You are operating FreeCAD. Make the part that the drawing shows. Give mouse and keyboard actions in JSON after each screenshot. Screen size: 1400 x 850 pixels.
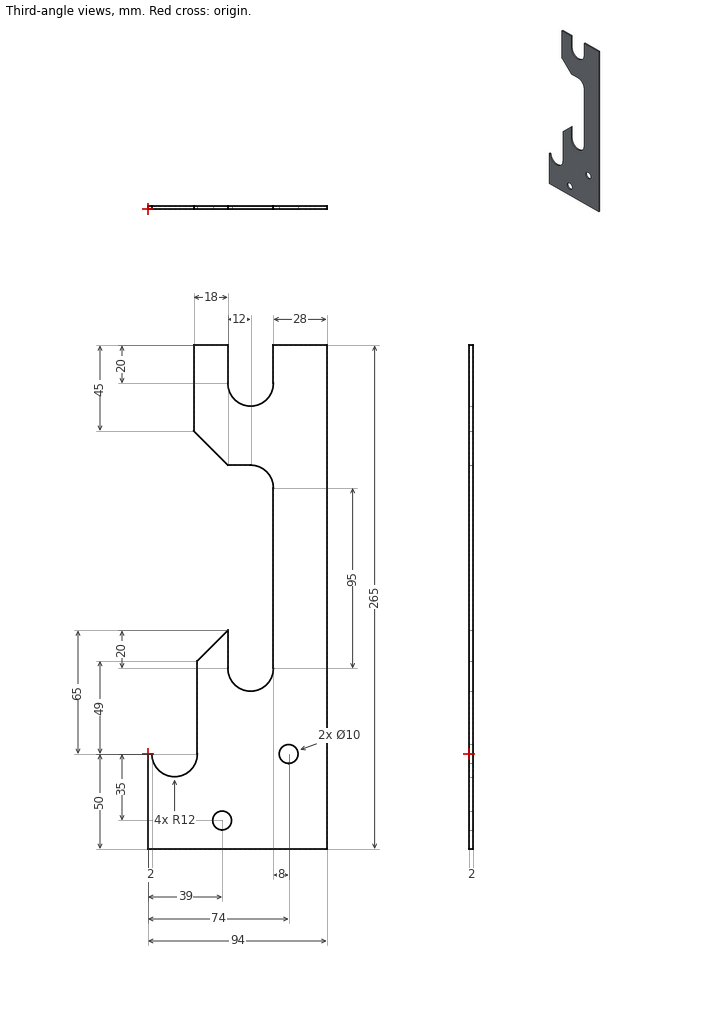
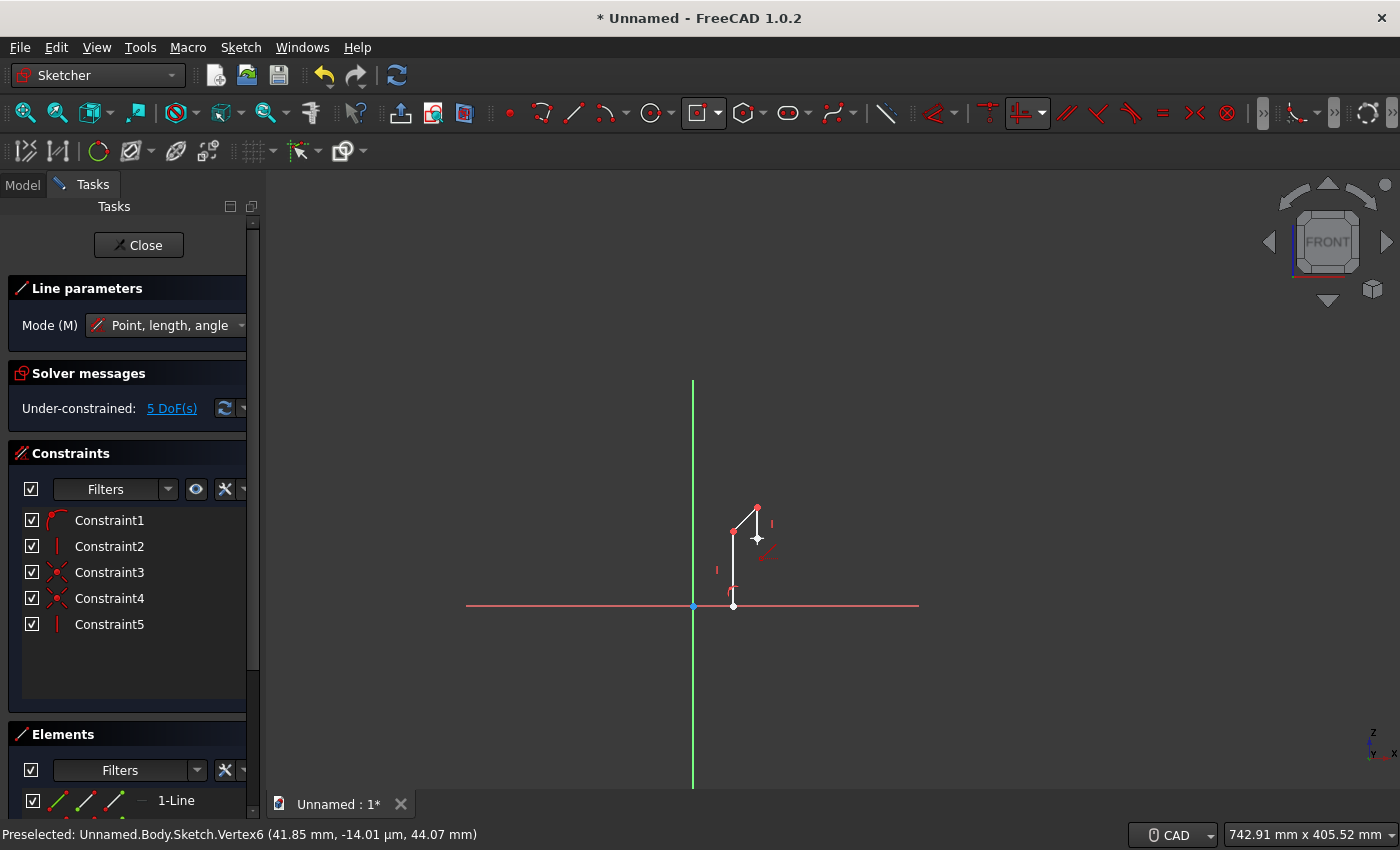
{"action": "left_click", "coordinate": [794, 538]}
{"action": "left_click", "coordinate": [794, 393]}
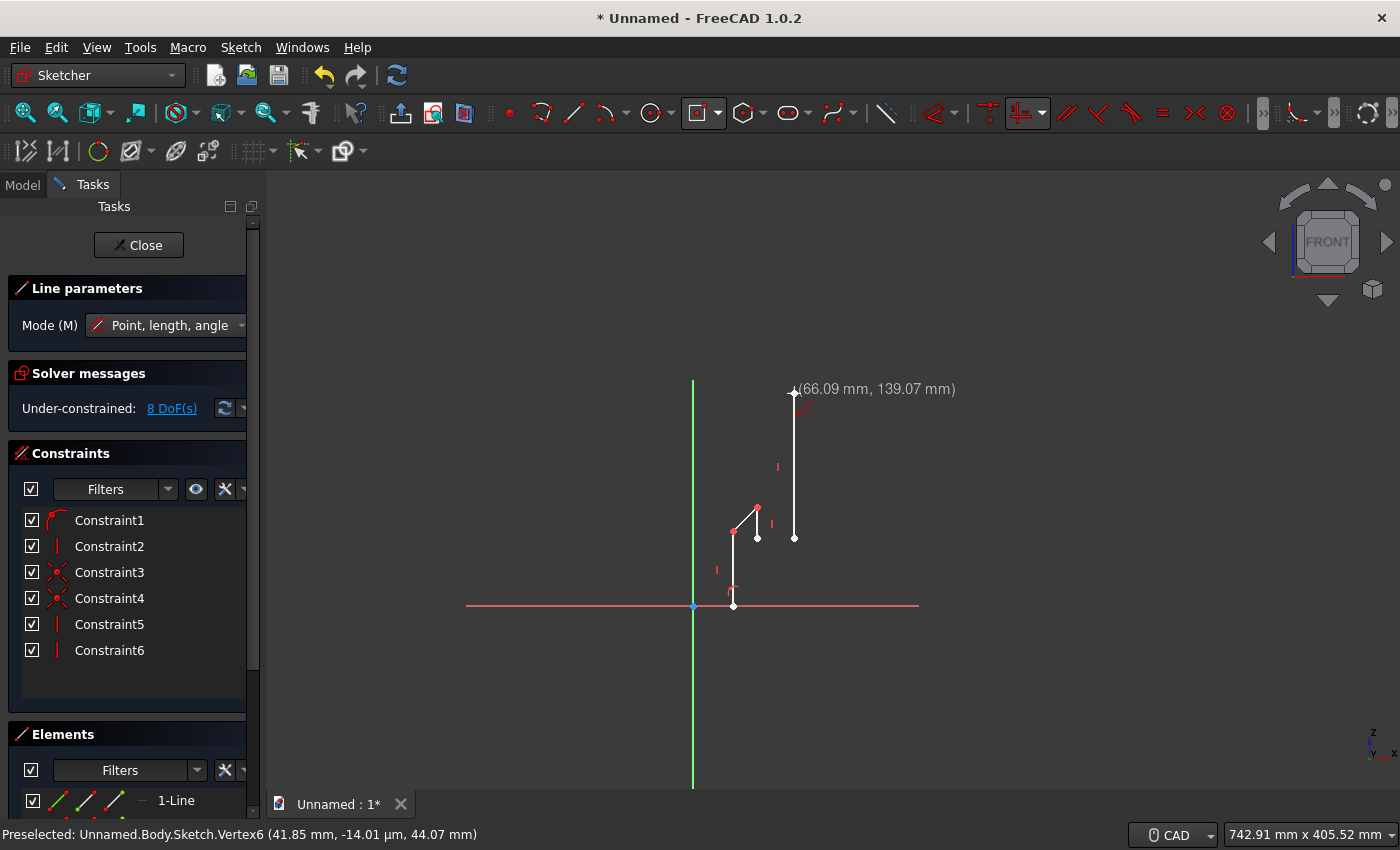
{"action": "left_click", "coordinate": [542, 114]}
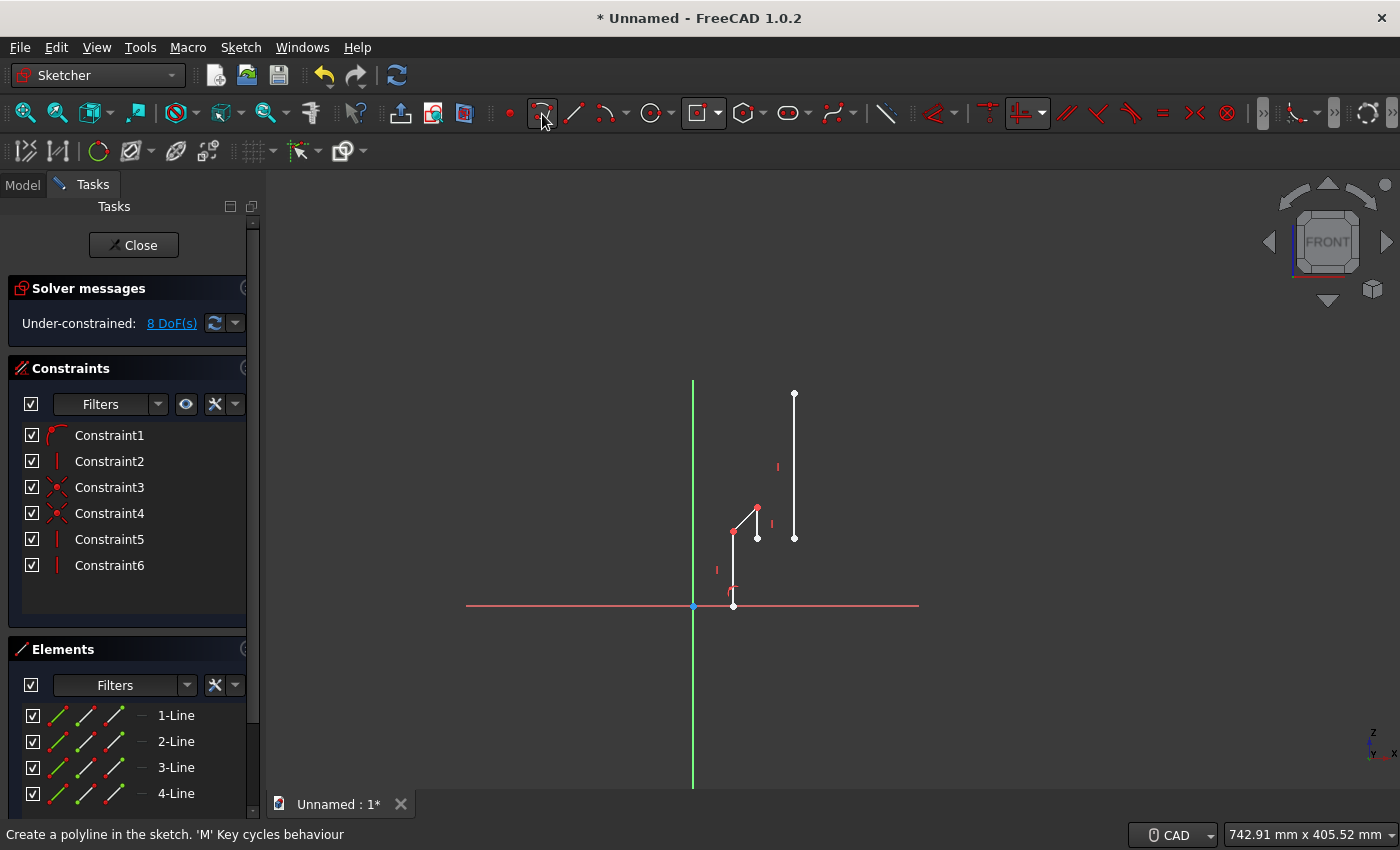
{"action": "left_click", "coordinate": [776, 374]}
{"action": "left_click", "coordinate": [757, 374]}
{"action": "left_click", "coordinate": [730, 347]}
{"action": "left_click", "coordinate": [730, 278]}
{"action": "left_click", "coordinate": [757, 278]}
{"action": "left_click", "coordinate": [757, 309]}
{"action": "right_click", "coordinate": [757, 309]}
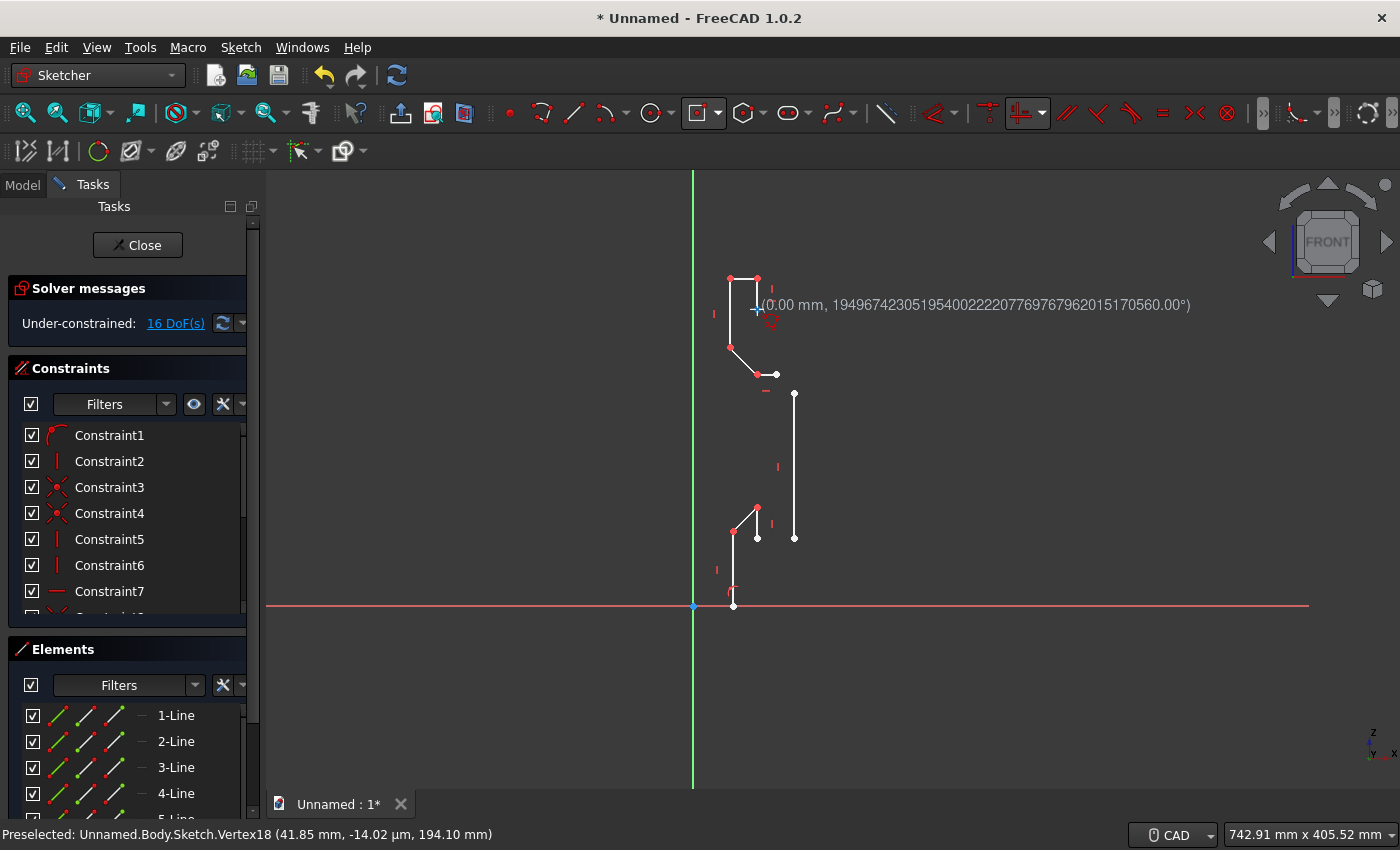
{"action": "left_click", "coordinate": [794, 309]}
{"action": "left_click", "coordinate": [794, 278]}
{"action": "left_click", "coordinate": [837, 278]}
{"action": "left_click", "coordinate": [837, 683]}
{"action": "left_click", "coordinate": [693, 683]}
{"action": "left_click", "coordinate": [693, 606]}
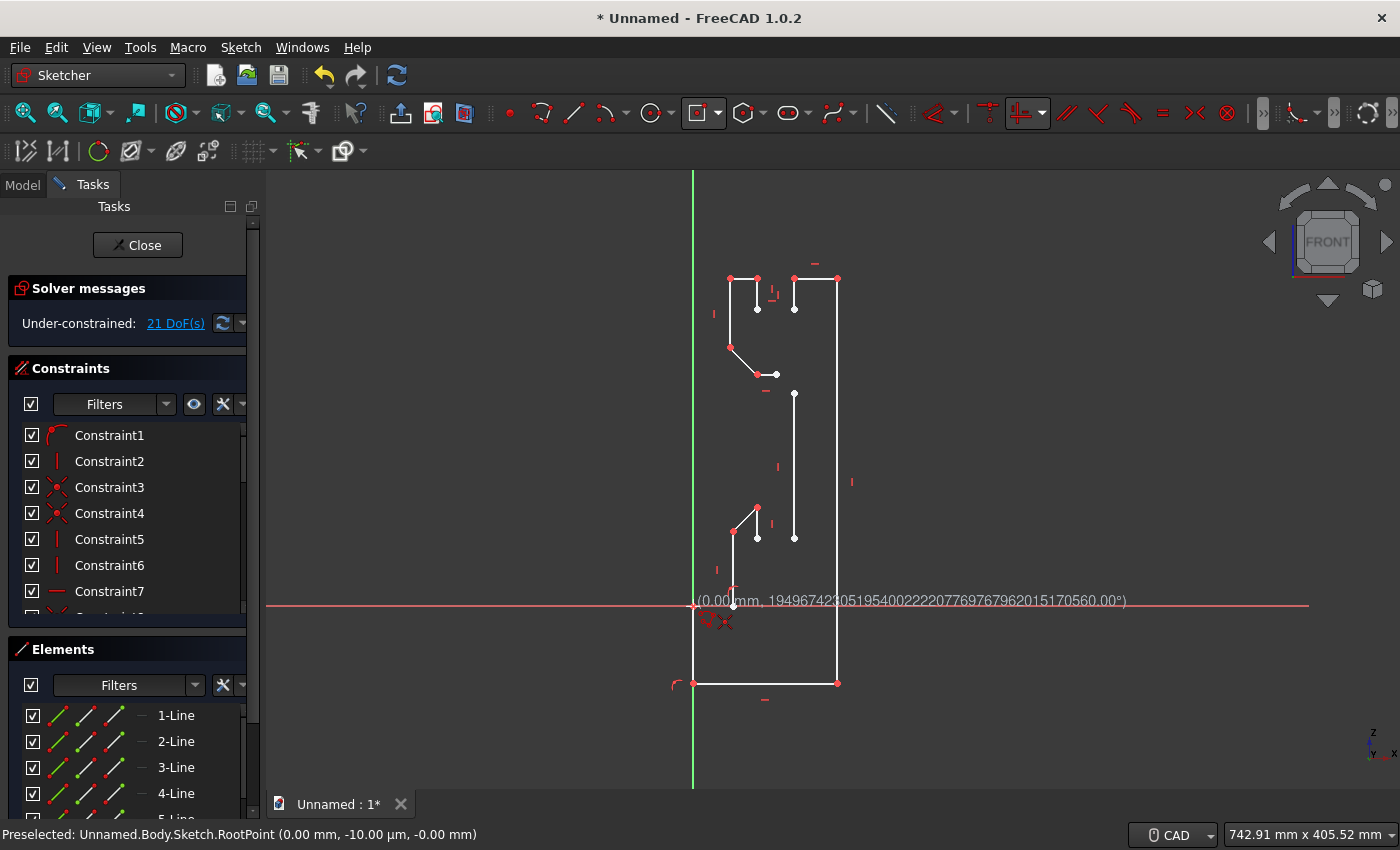
{"action": "scroll", "coordinate": [696, 606], "scroll_direction": "up", "scroll_amount": 9}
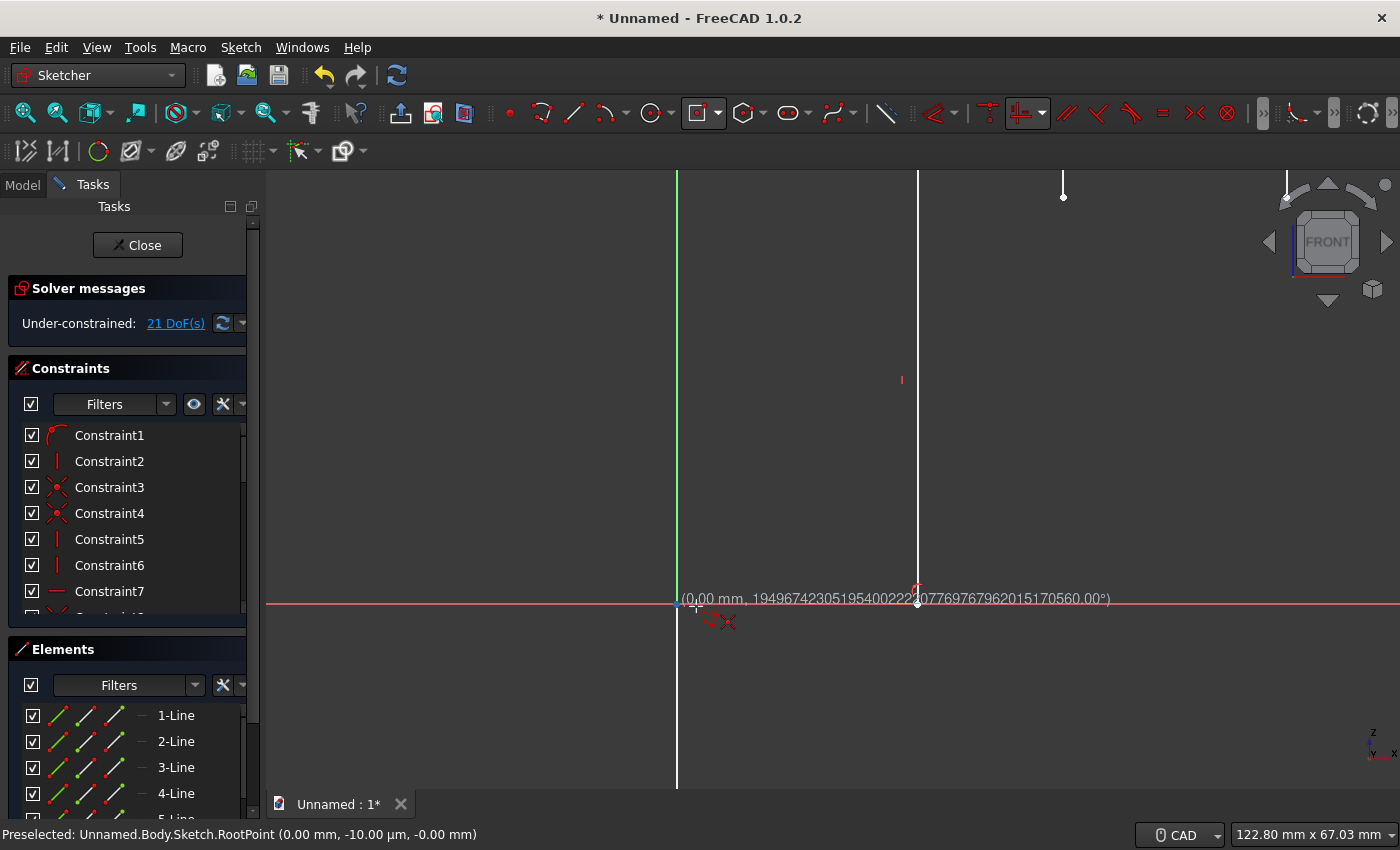
{"action": "left_click", "coordinate": [695, 595]}
{"action": "right_click", "coordinate": [695, 595]}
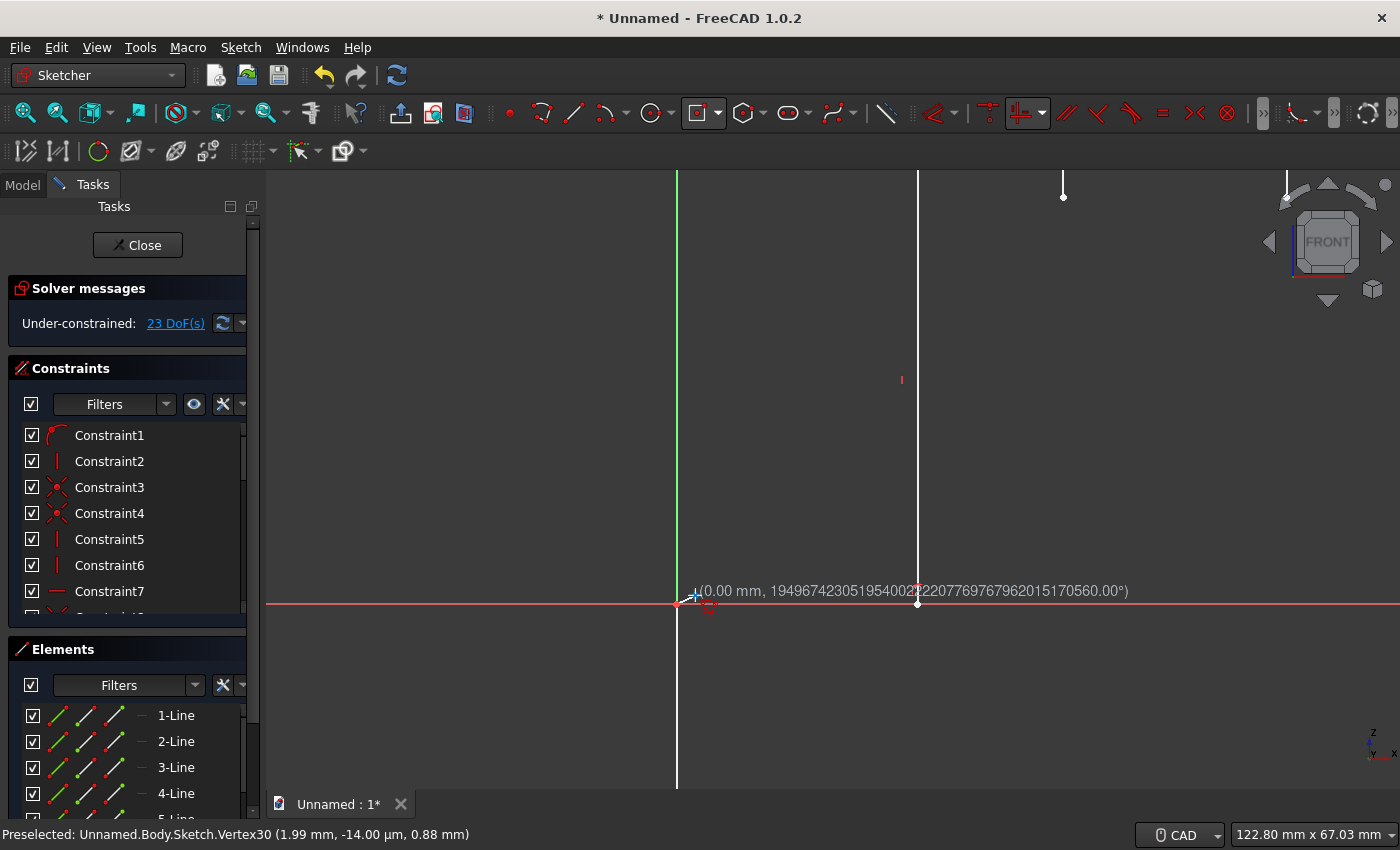
{"action": "key", "text": "g 3 a"}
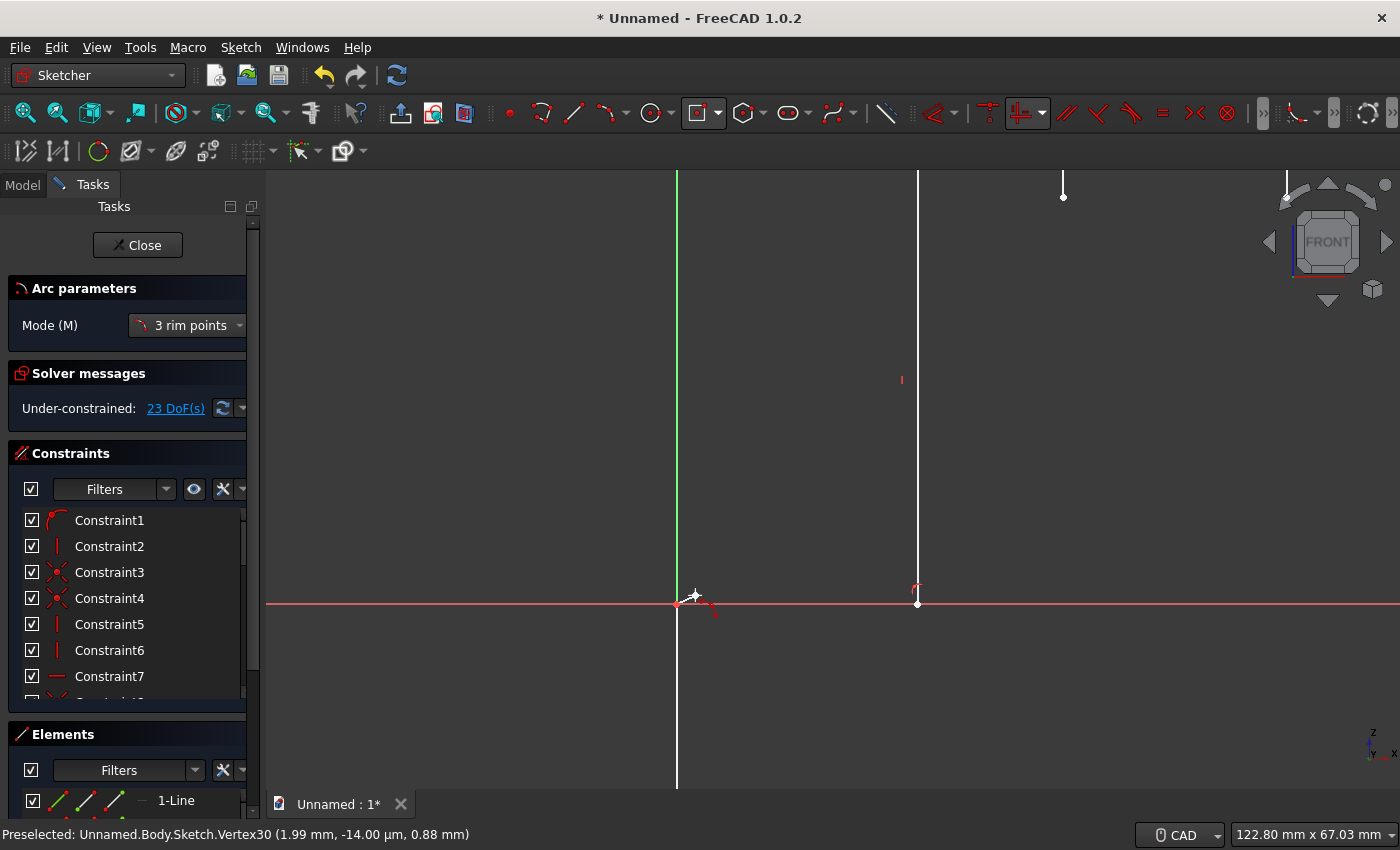
{"action": "scroll", "coordinate": [696, 606], "scroll_direction": "down", "scroll_amount": 9}